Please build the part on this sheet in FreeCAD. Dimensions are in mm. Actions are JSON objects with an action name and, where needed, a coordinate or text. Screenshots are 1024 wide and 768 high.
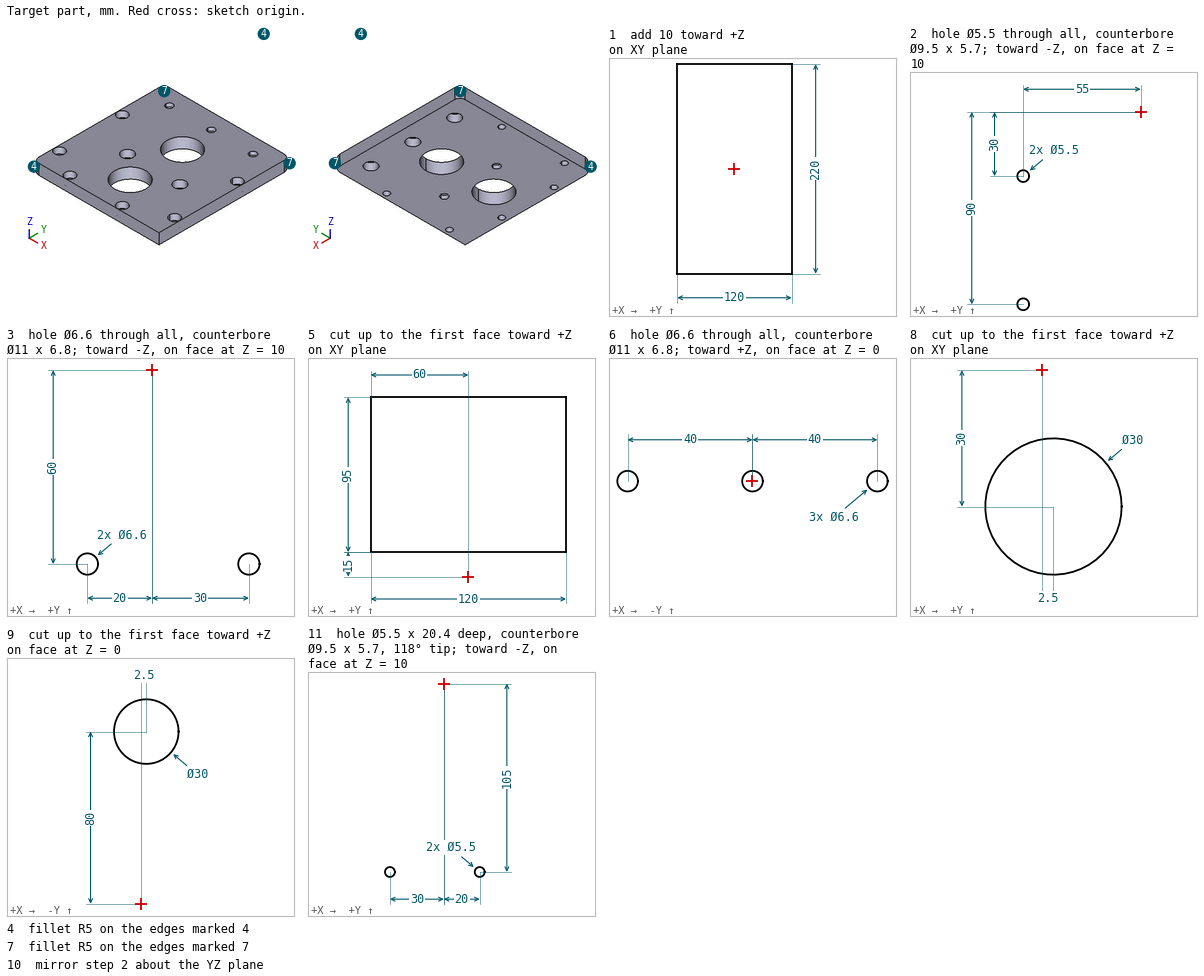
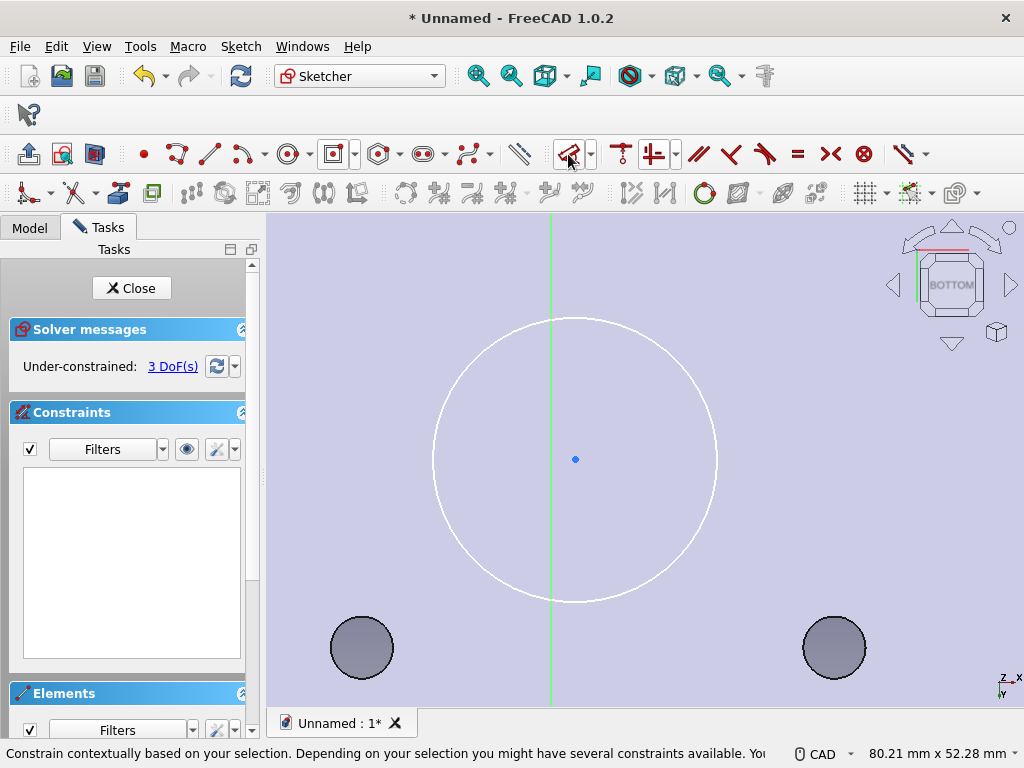
{"action": "left_click", "coordinate": [675, 359]}
{"action": "left_click", "coordinate": [698, 336]}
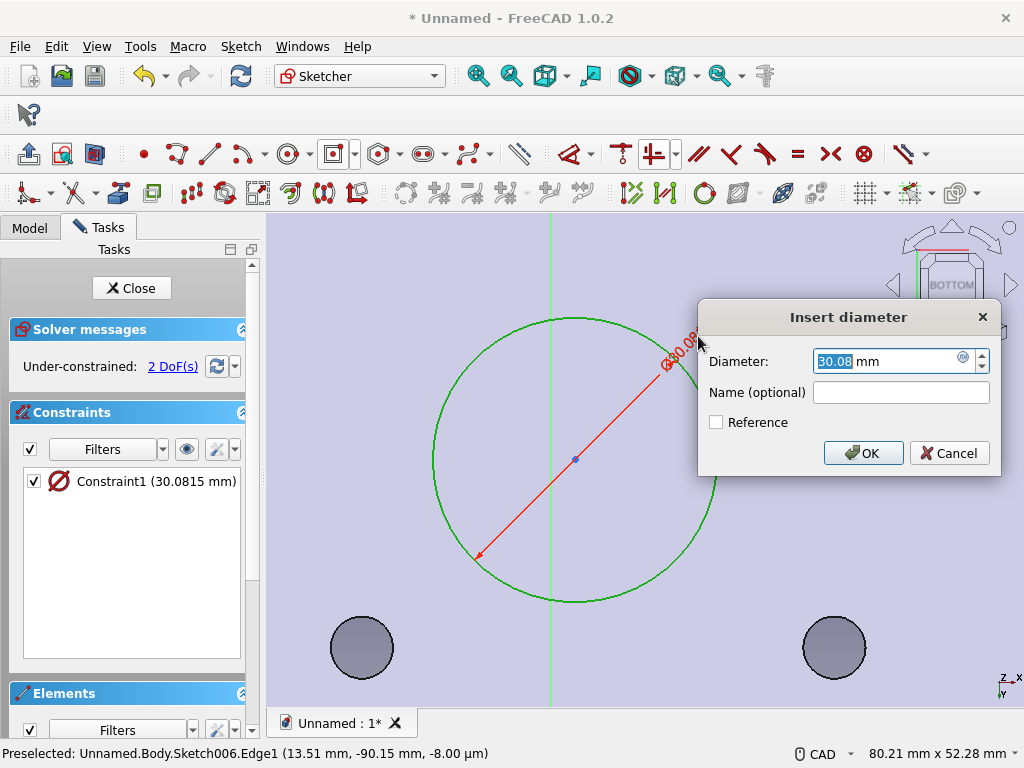
{"action": "type", "text": "30"}
{"action": "key", "text": "Return"}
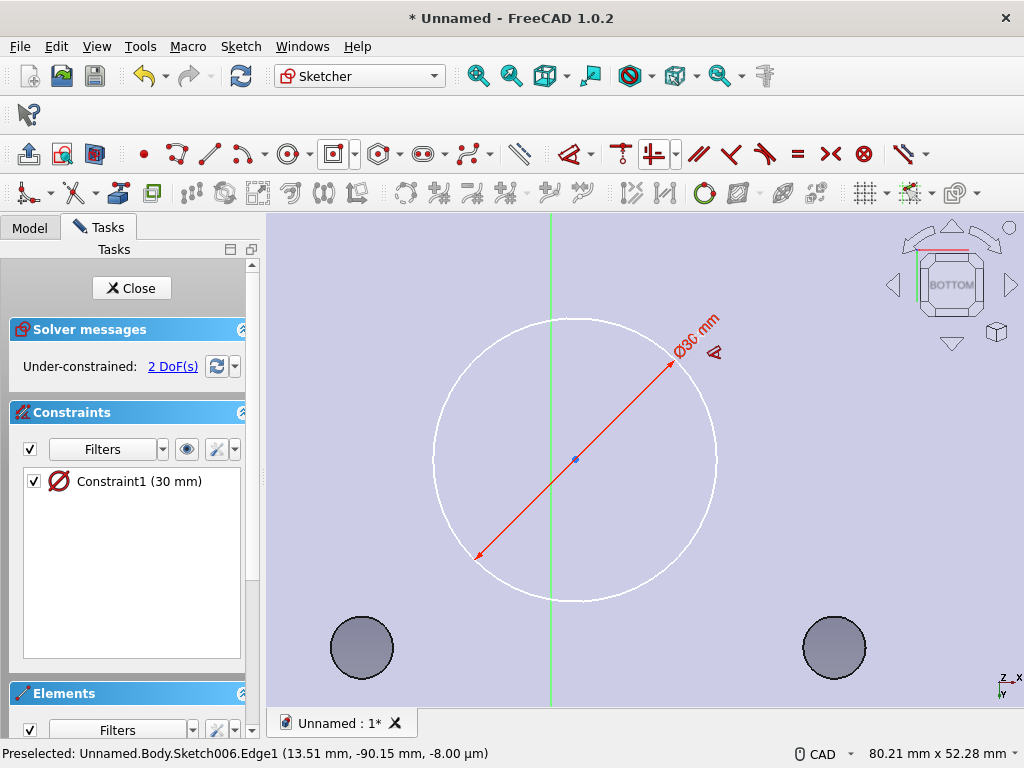
{"action": "left_click", "coordinate": [575, 460]}
{"action": "left_click", "coordinate": [517, 570]}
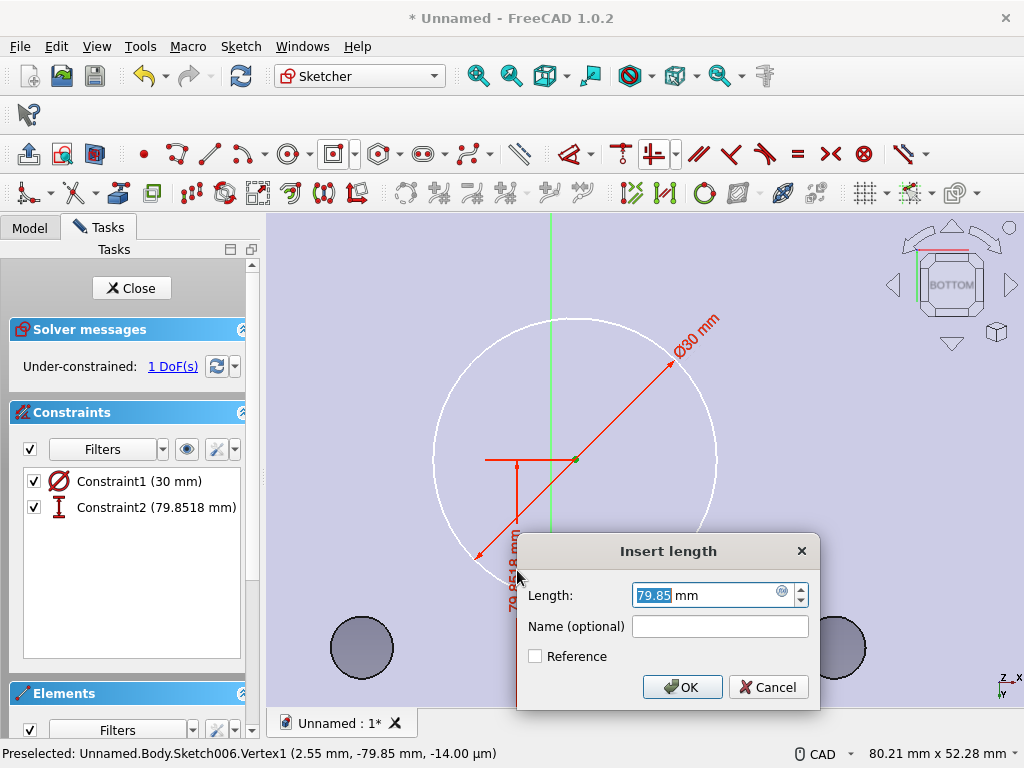
{"action": "type", "text": "80"}
{"action": "key", "text": "Return"}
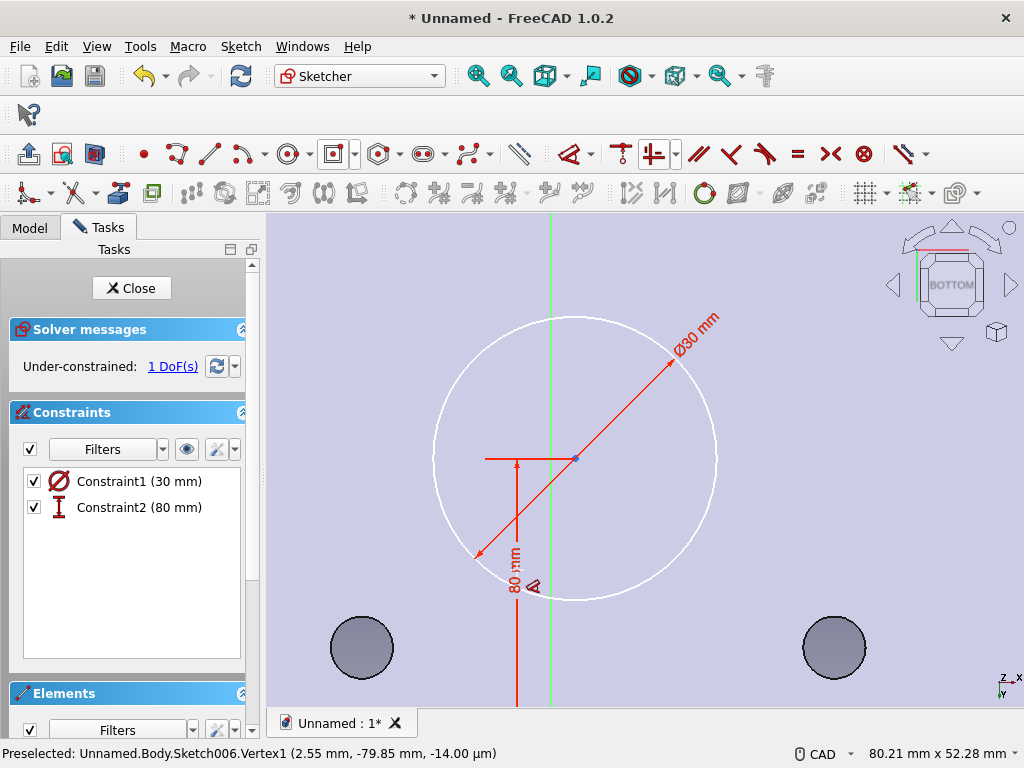
{"action": "scroll", "coordinate": [575, 459], "scroll_direction": "up", "scroll_amount": 3}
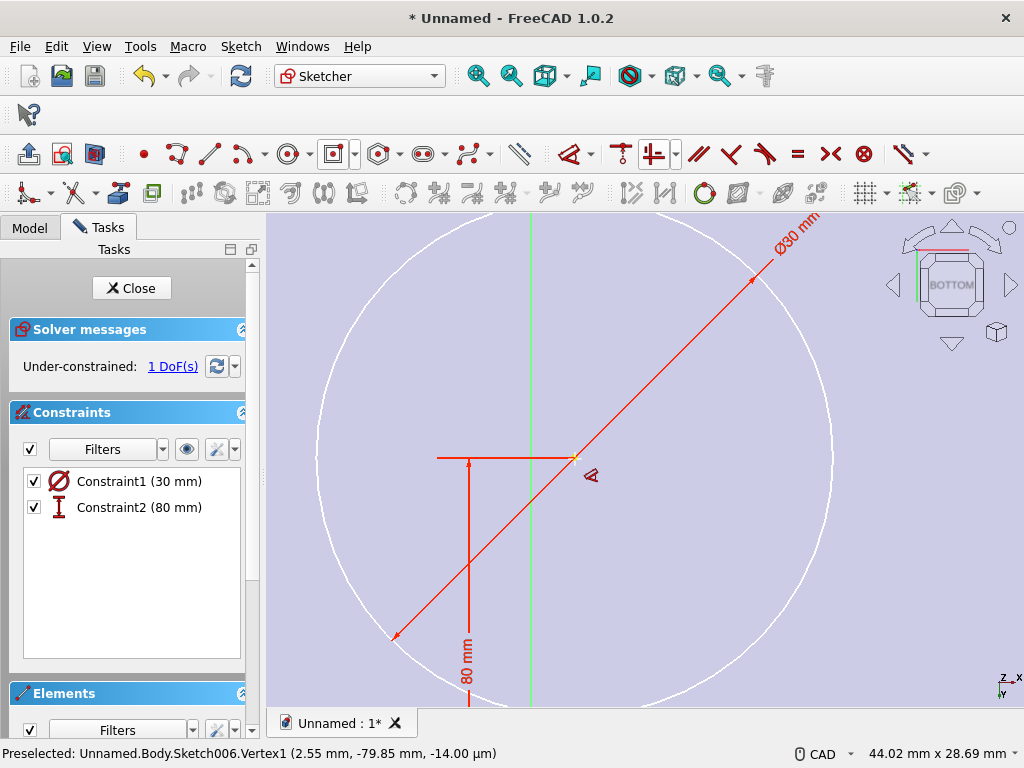
{"action": "left_click", "coordinate": [575, 458]}
{"action": "left_click", "coordinate": [553, 424]}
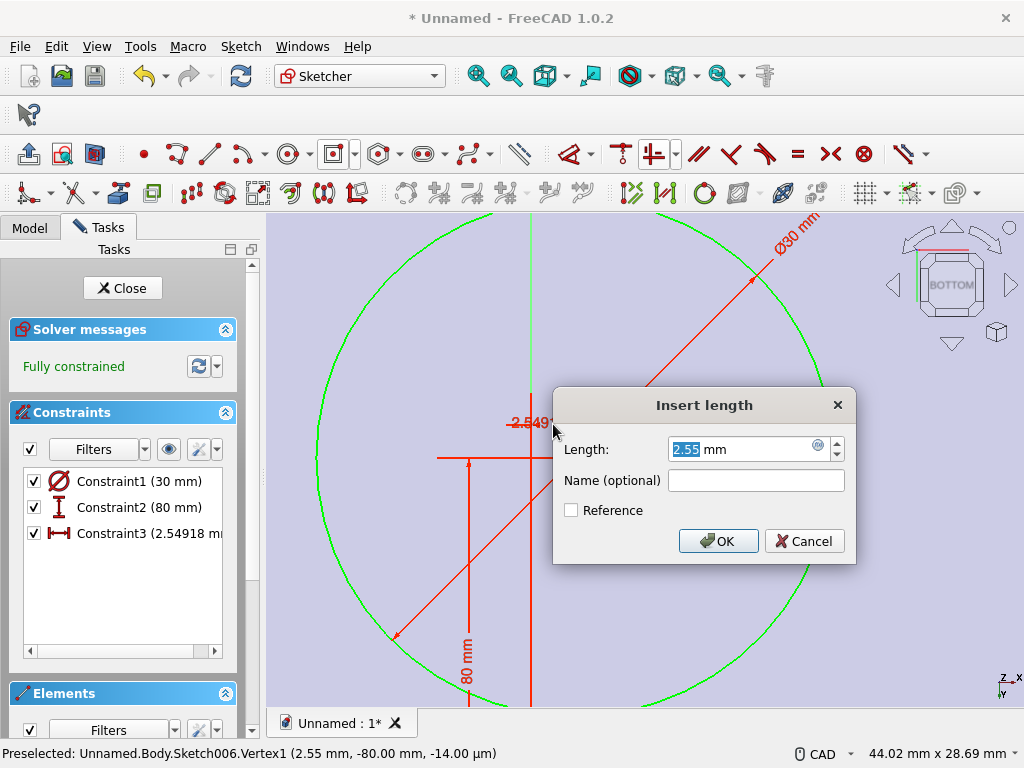
{"action": "type", "text": "2.5"}
{"action": "key", "text": "Return"}
{"action": "key", "text": "Escape"}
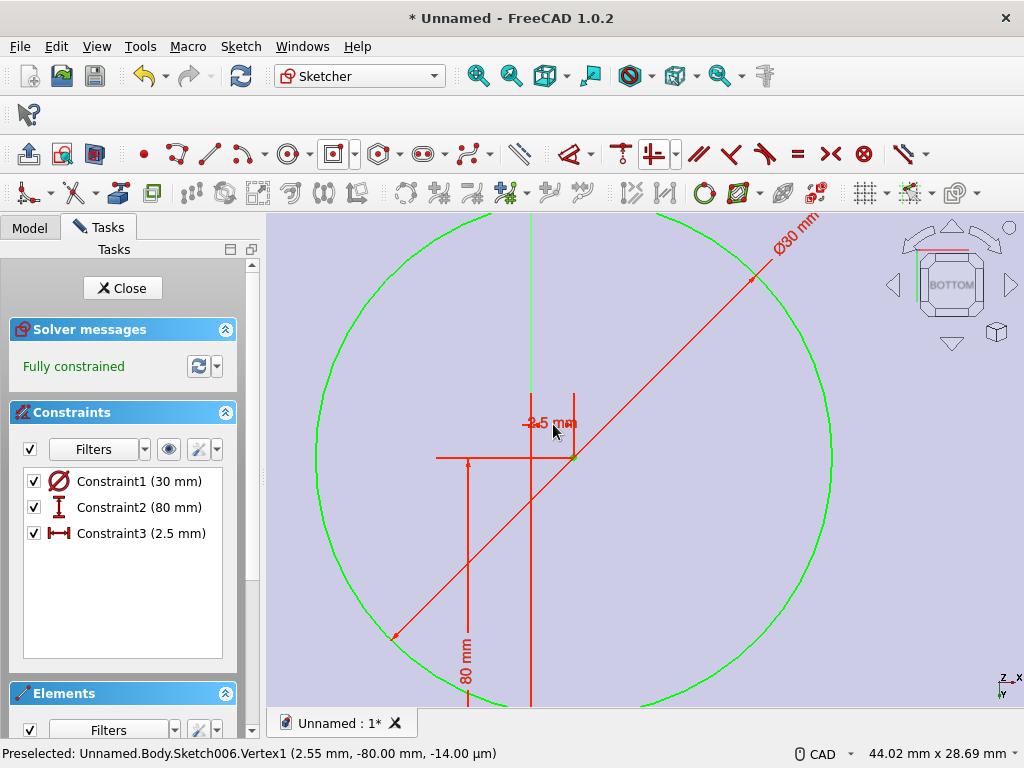
{"action": "left_click", "coordinate": [123, 288]}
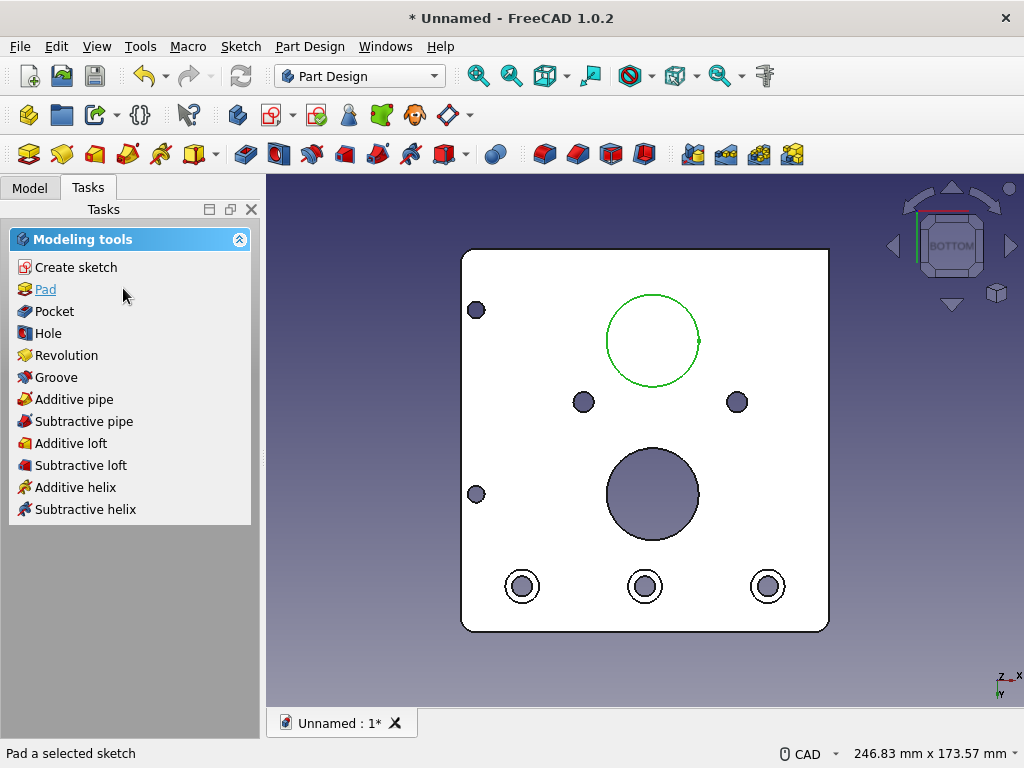
{"action": "left_click", "coordinate": [246, 154]}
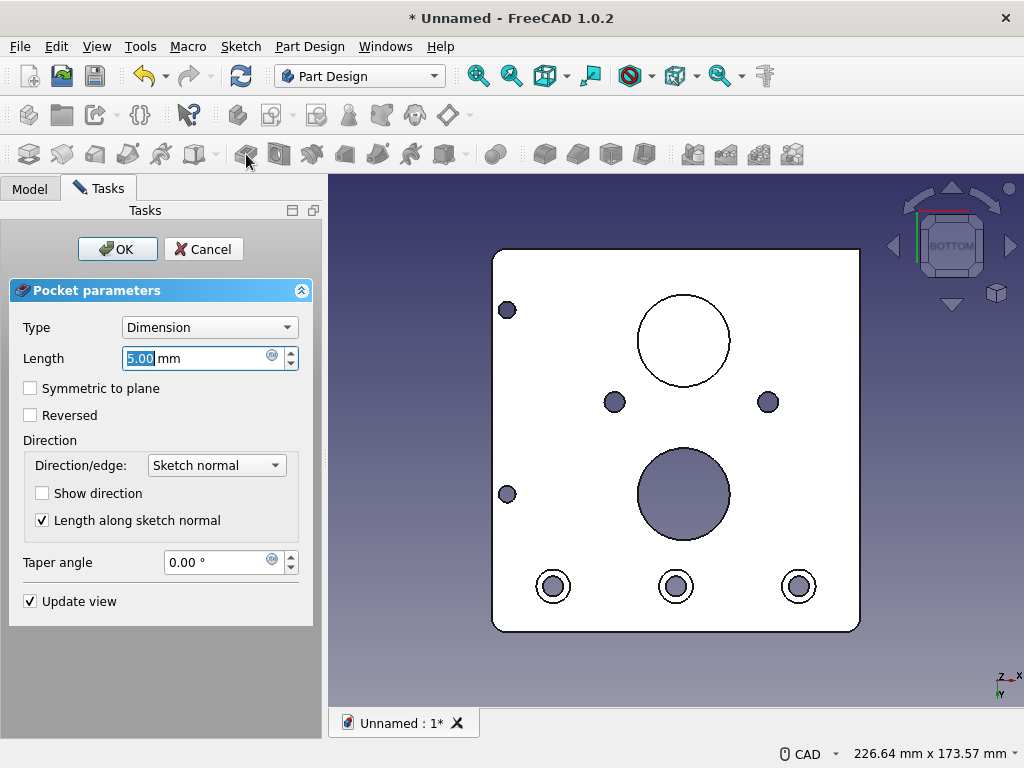
{"action": "left_click", "coordinate": [210, 328]}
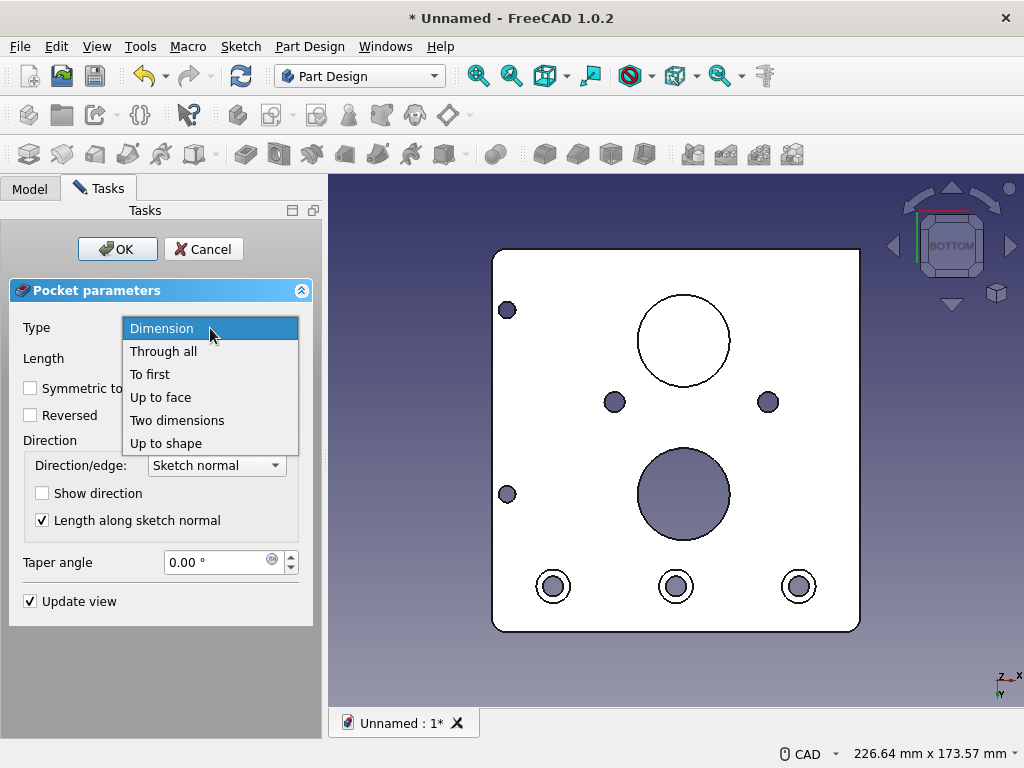
{"action": "left_click", "coordinate": [208, 374]}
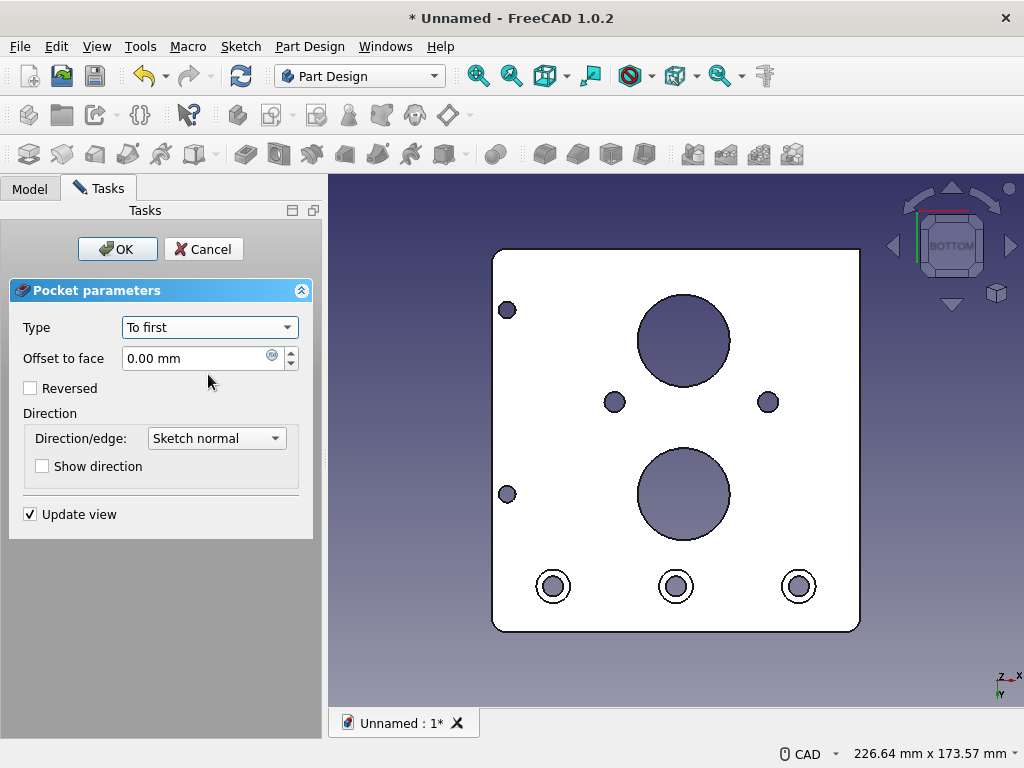
{"action": "left_click", "coordinate": [118, 249]}